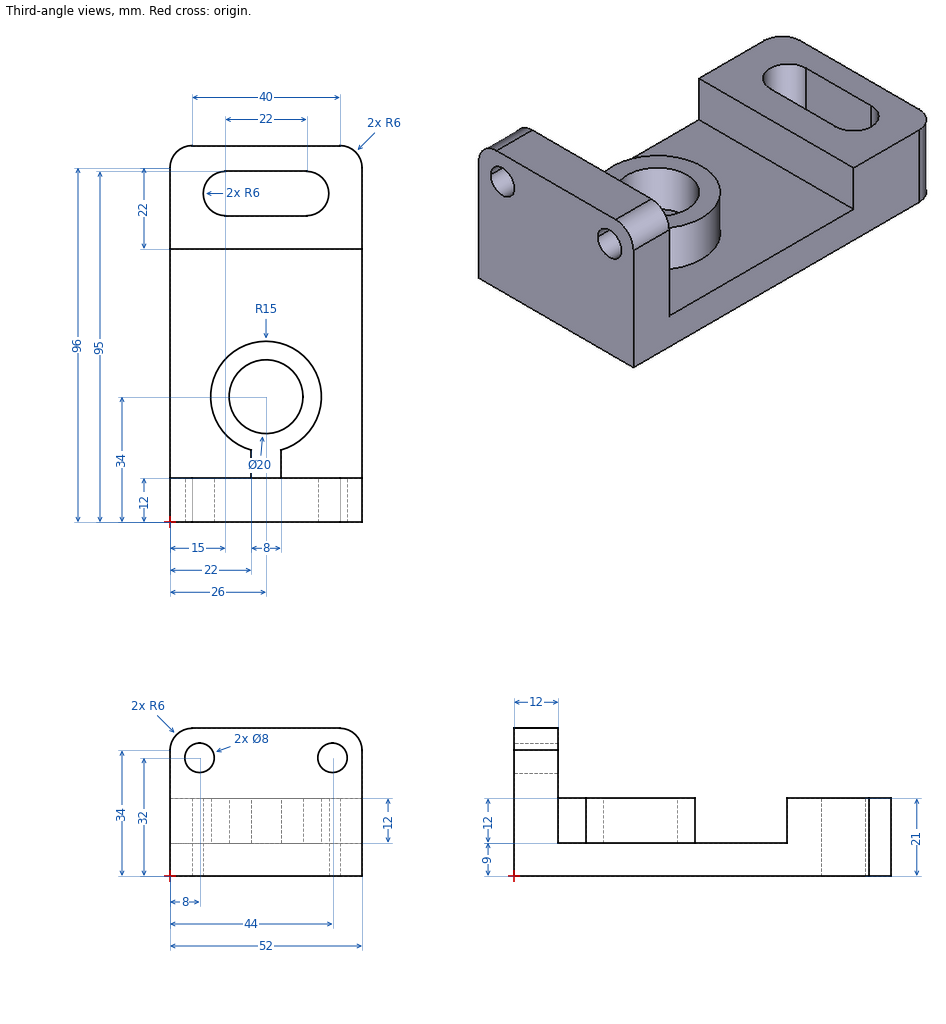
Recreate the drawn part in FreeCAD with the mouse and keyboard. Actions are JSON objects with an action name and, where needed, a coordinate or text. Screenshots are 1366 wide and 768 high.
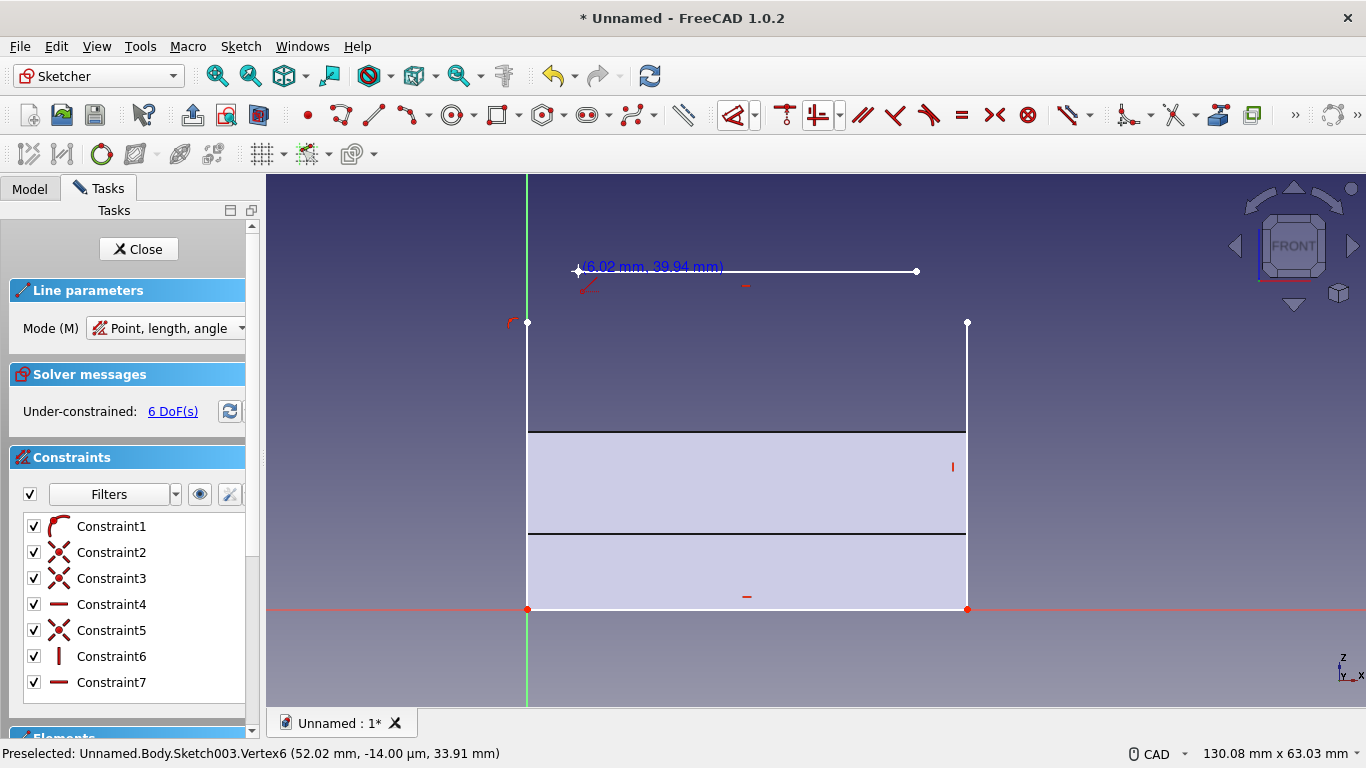
{"action": "left_click", "coordinate": [406, 116]}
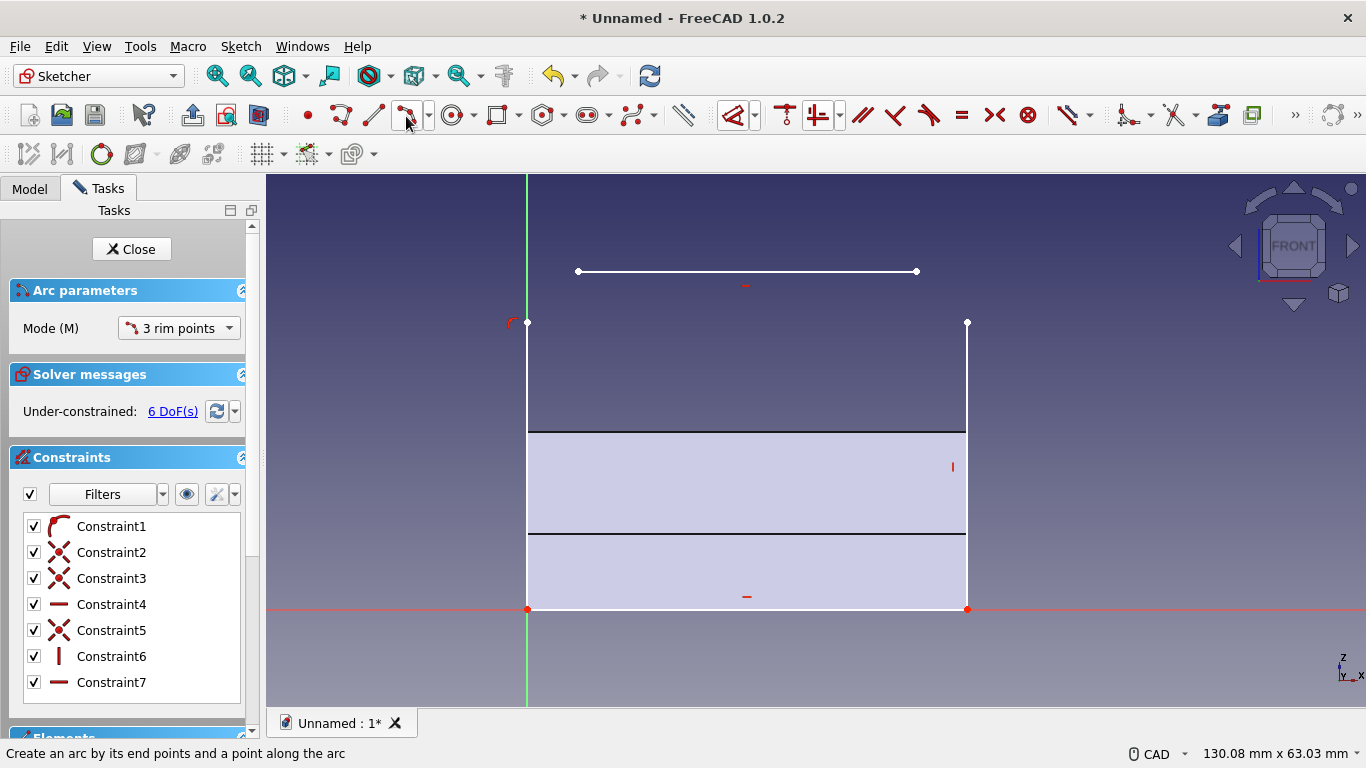
{"action": "left_click", "coordinate": [967, 323]}
{"action": "left_click", "coordinate": [916, 272]}
{"action": "left_click", "coordinate": [952, 286]}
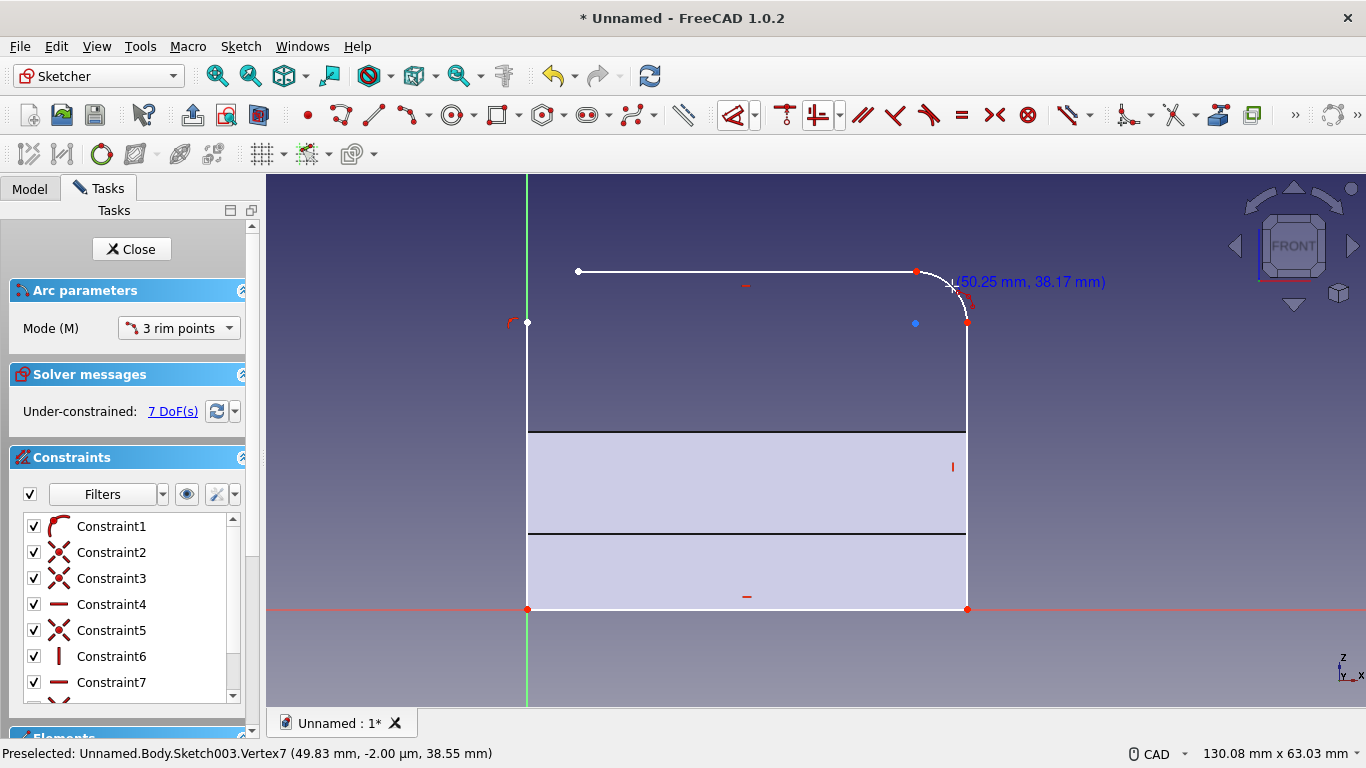
{"action": "left_click", "coordinate": [578, 272]}
{"action": "left_click", "coordinate": [527, 323]}
{"action": "left_click", "coordinate": [542, 286]}
{"action": "key", "text": "Escape"}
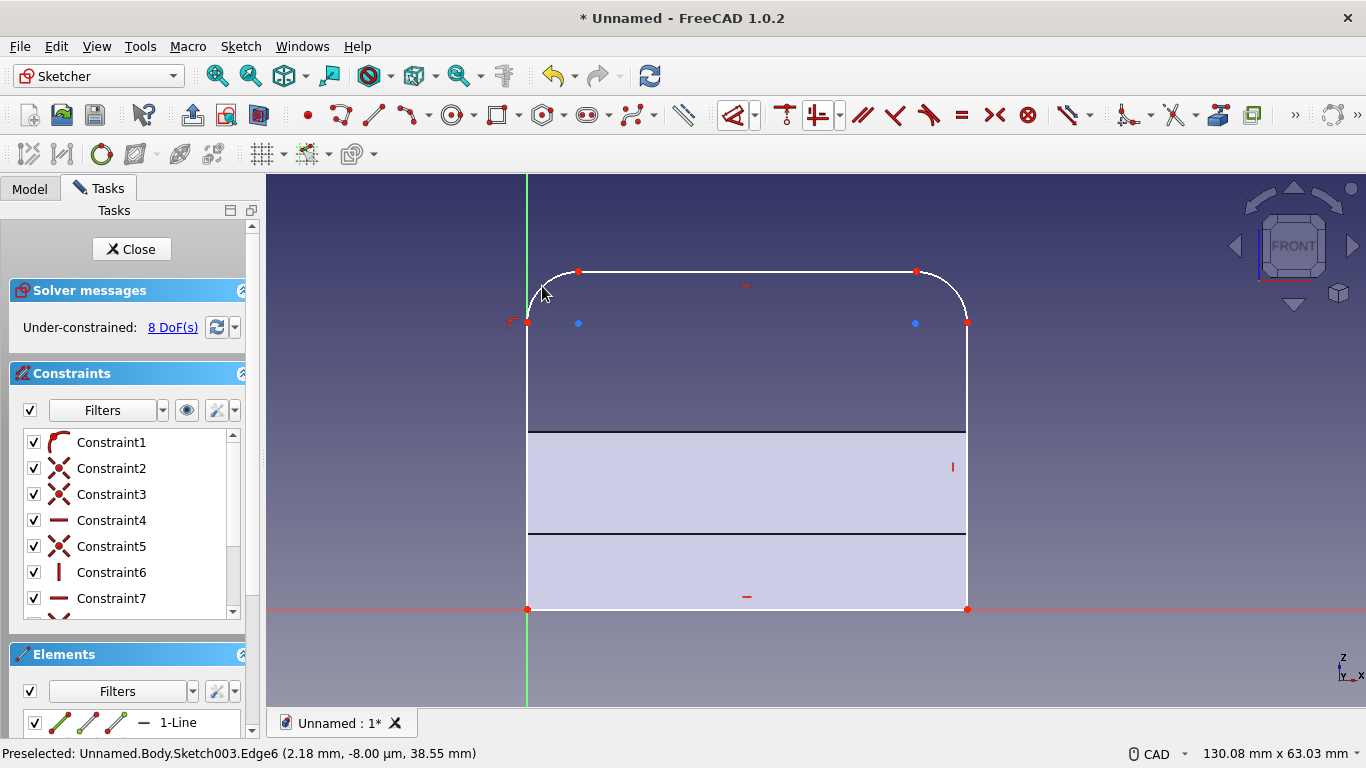
{"action": "left_click", "coordinate": [527, 409]}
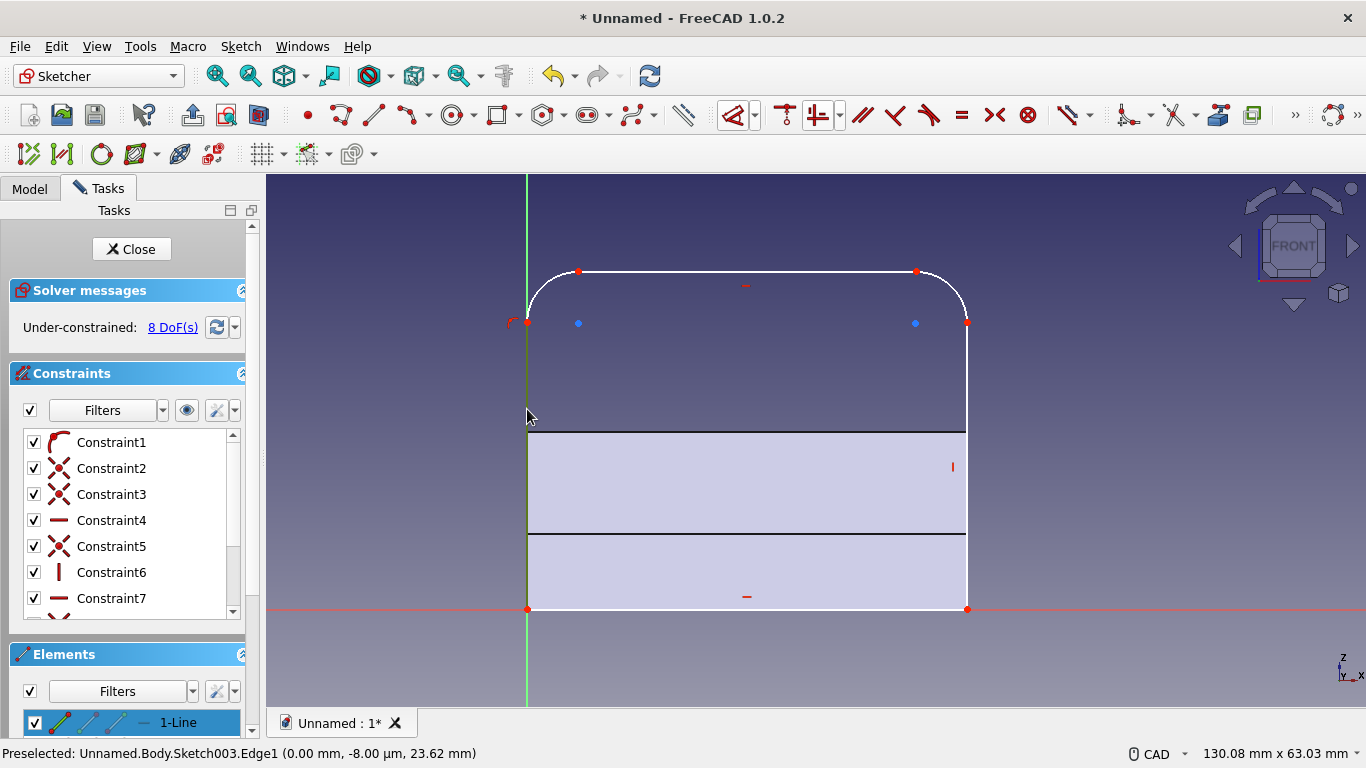
{"action": "left_click", "coordinate": [555, 278]}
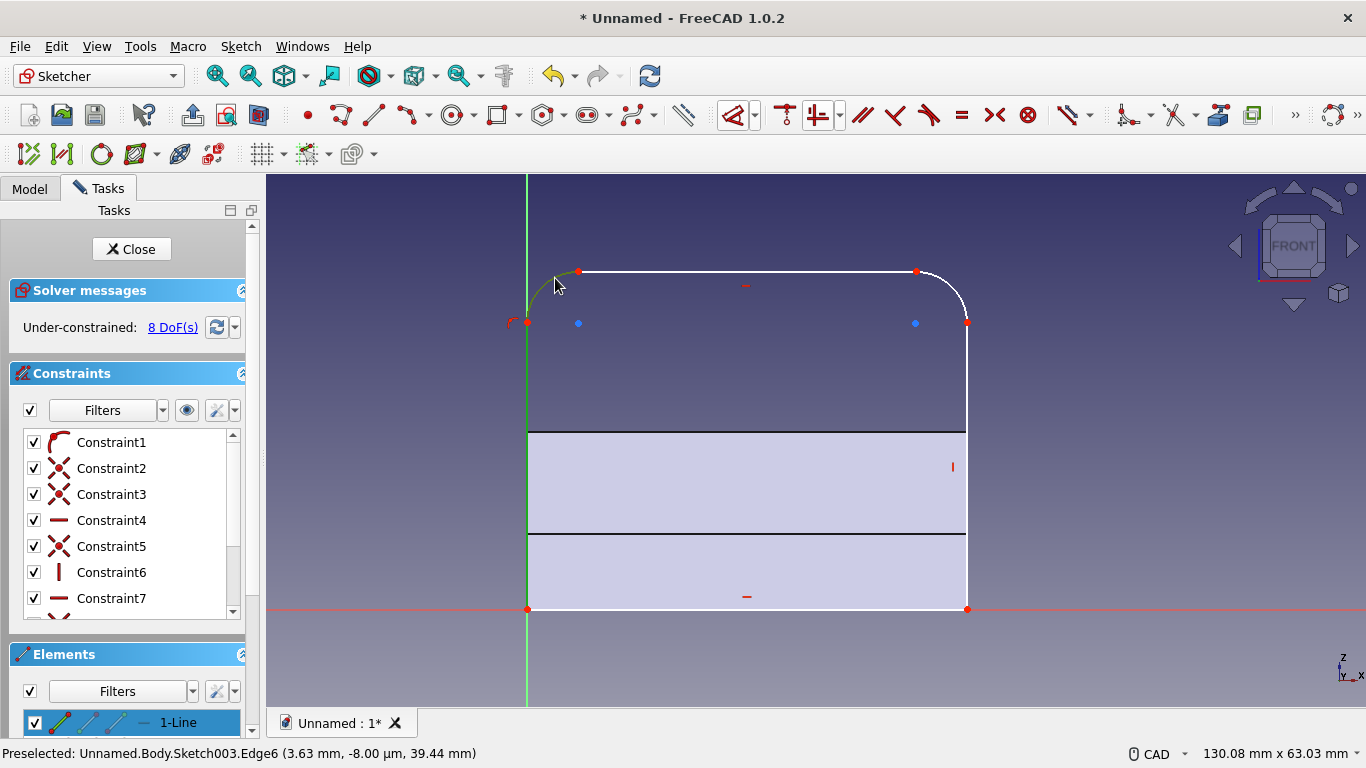
{"action": "key", "text": "t"}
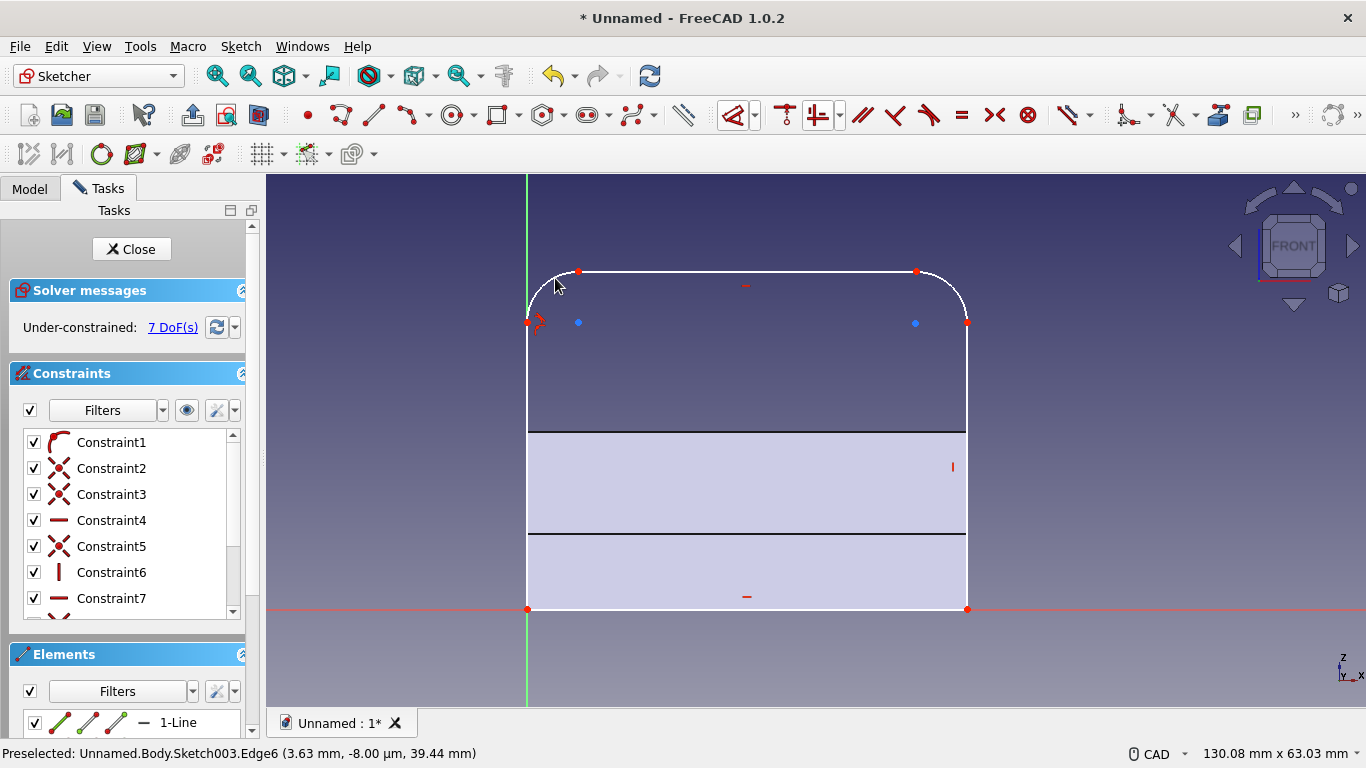
{"action": "left_click", "coordinate": [967, 524]}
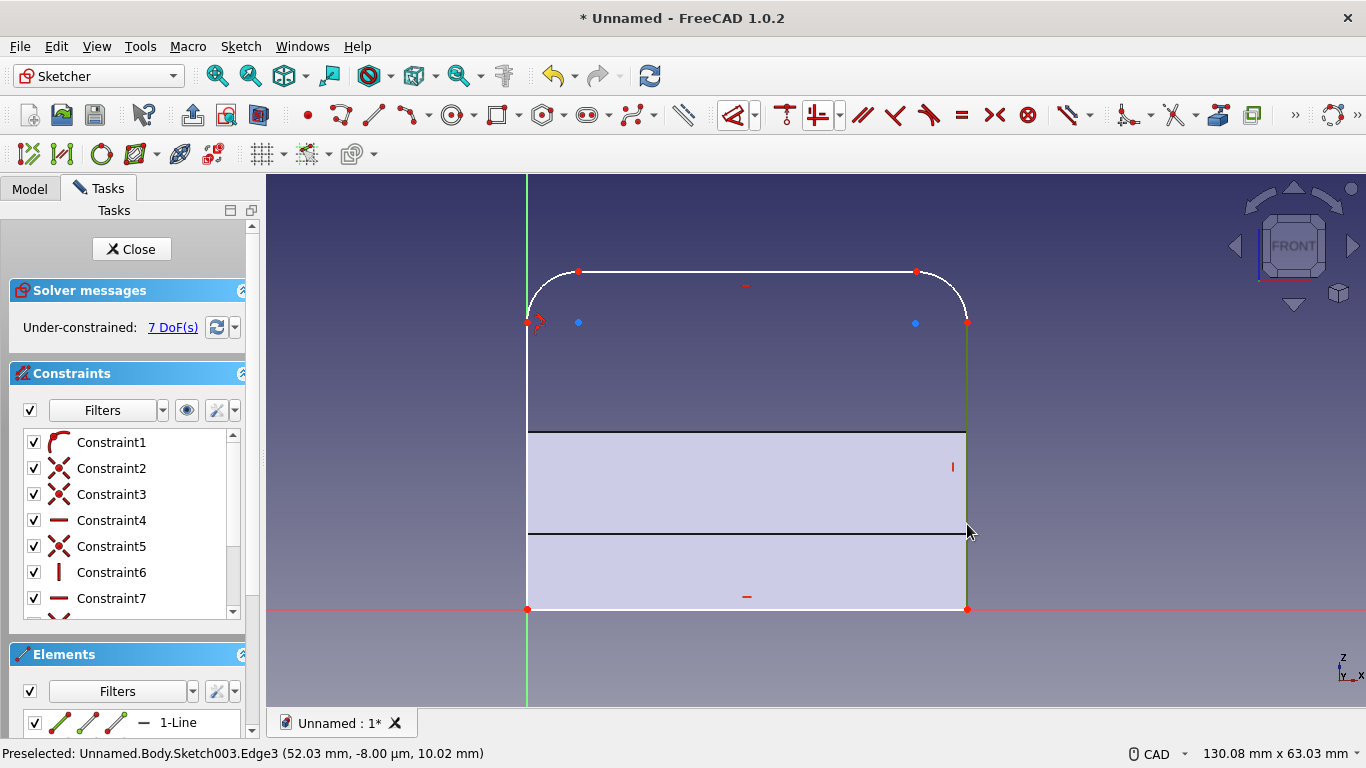
{"action": "left_click", "coordinate": [961, 300]}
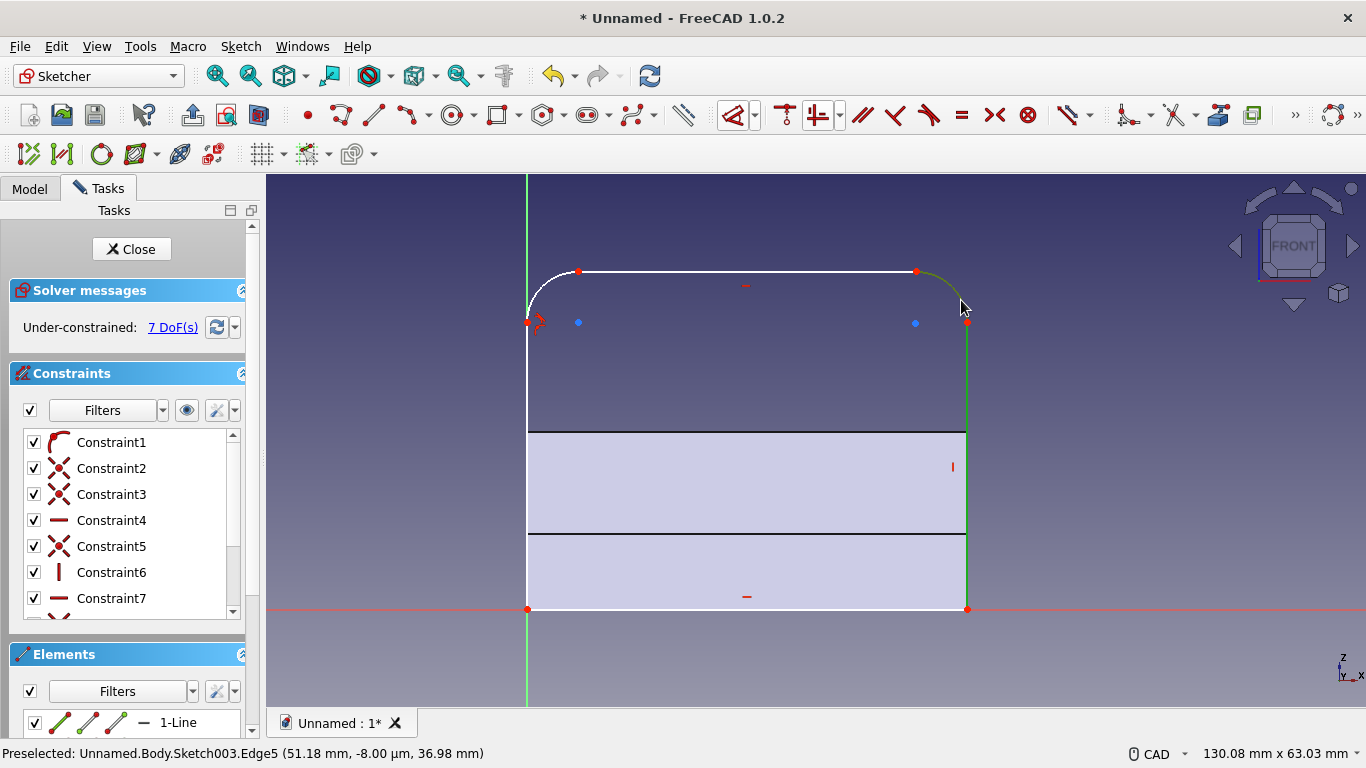
{"action": "left_click", "coordinate": [929, 116]}